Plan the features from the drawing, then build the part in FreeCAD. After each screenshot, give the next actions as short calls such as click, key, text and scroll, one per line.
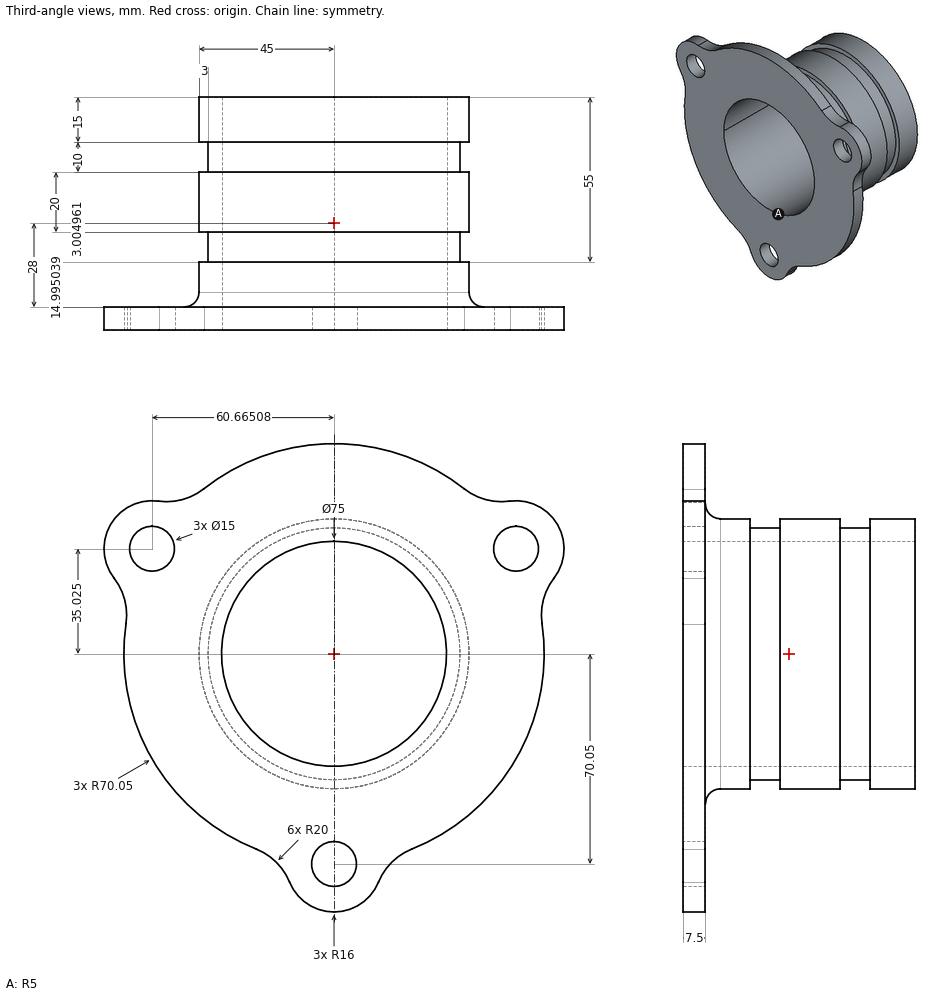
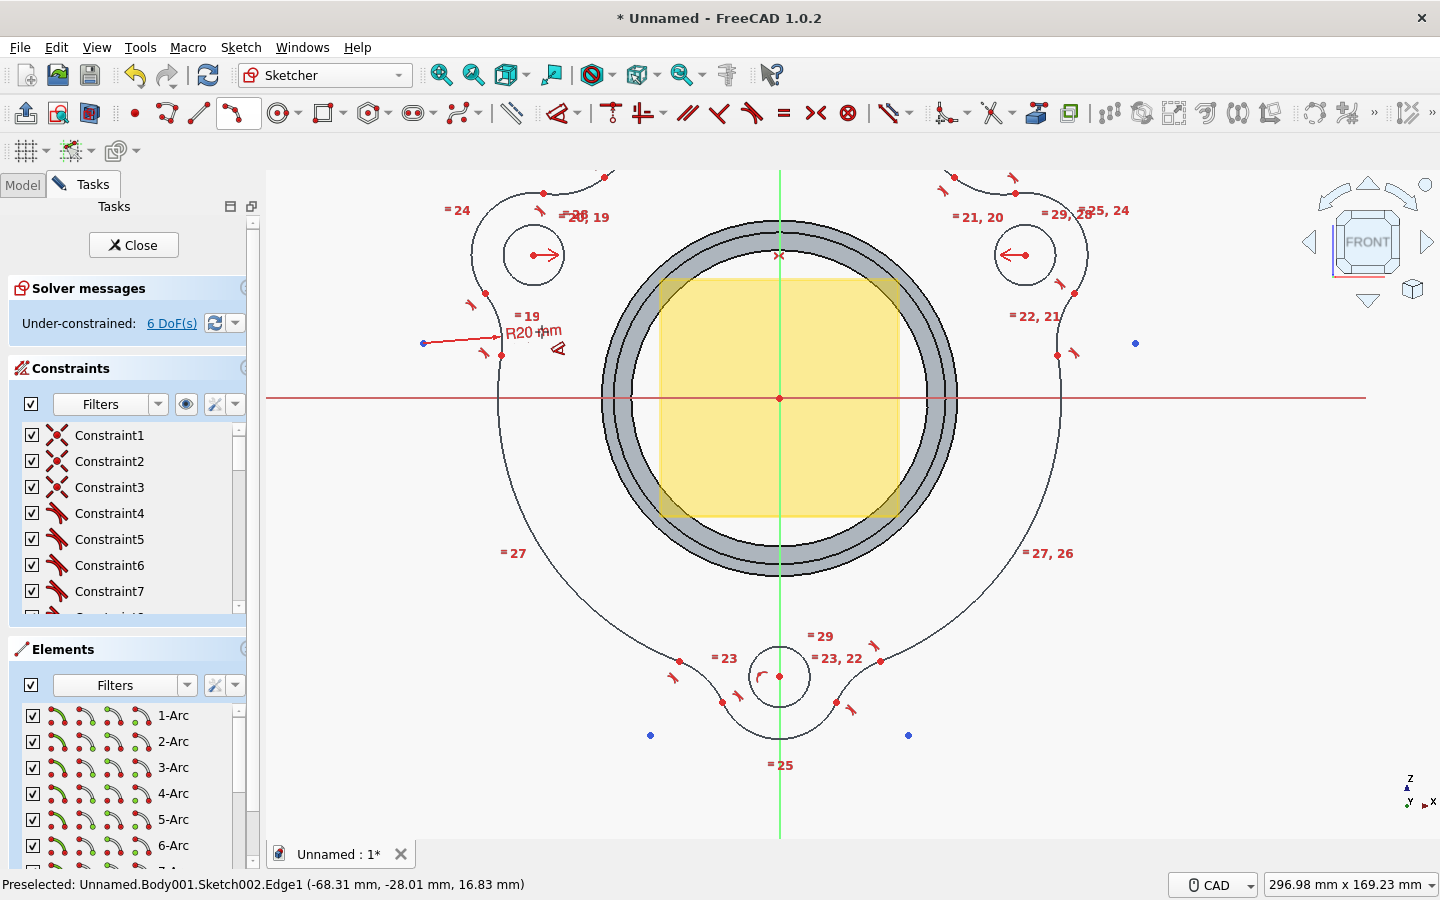
click(500, 202)
click(451, 209)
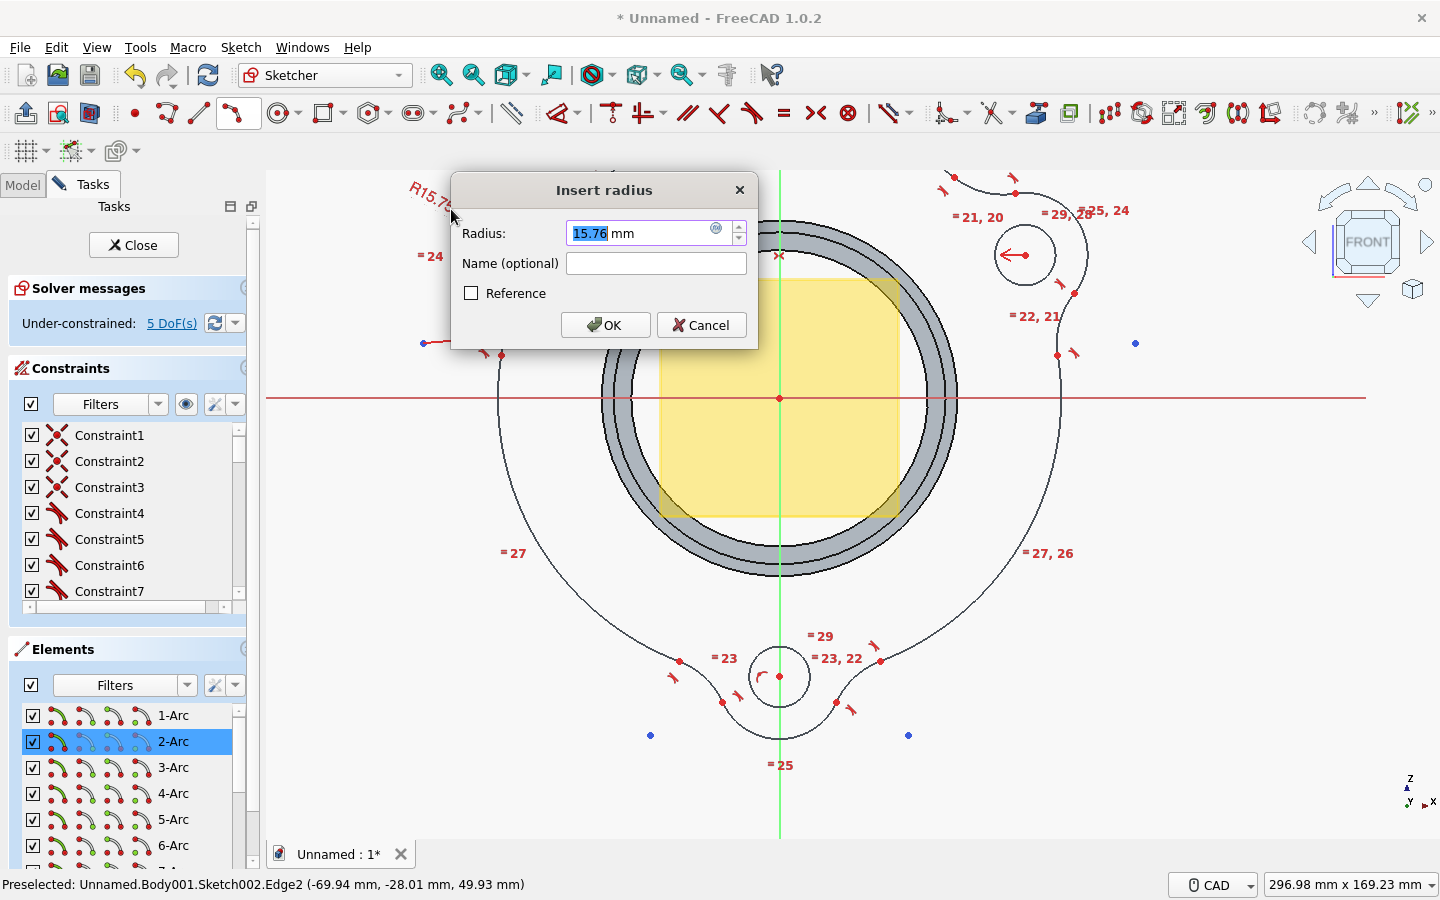
text(16)
key(Return)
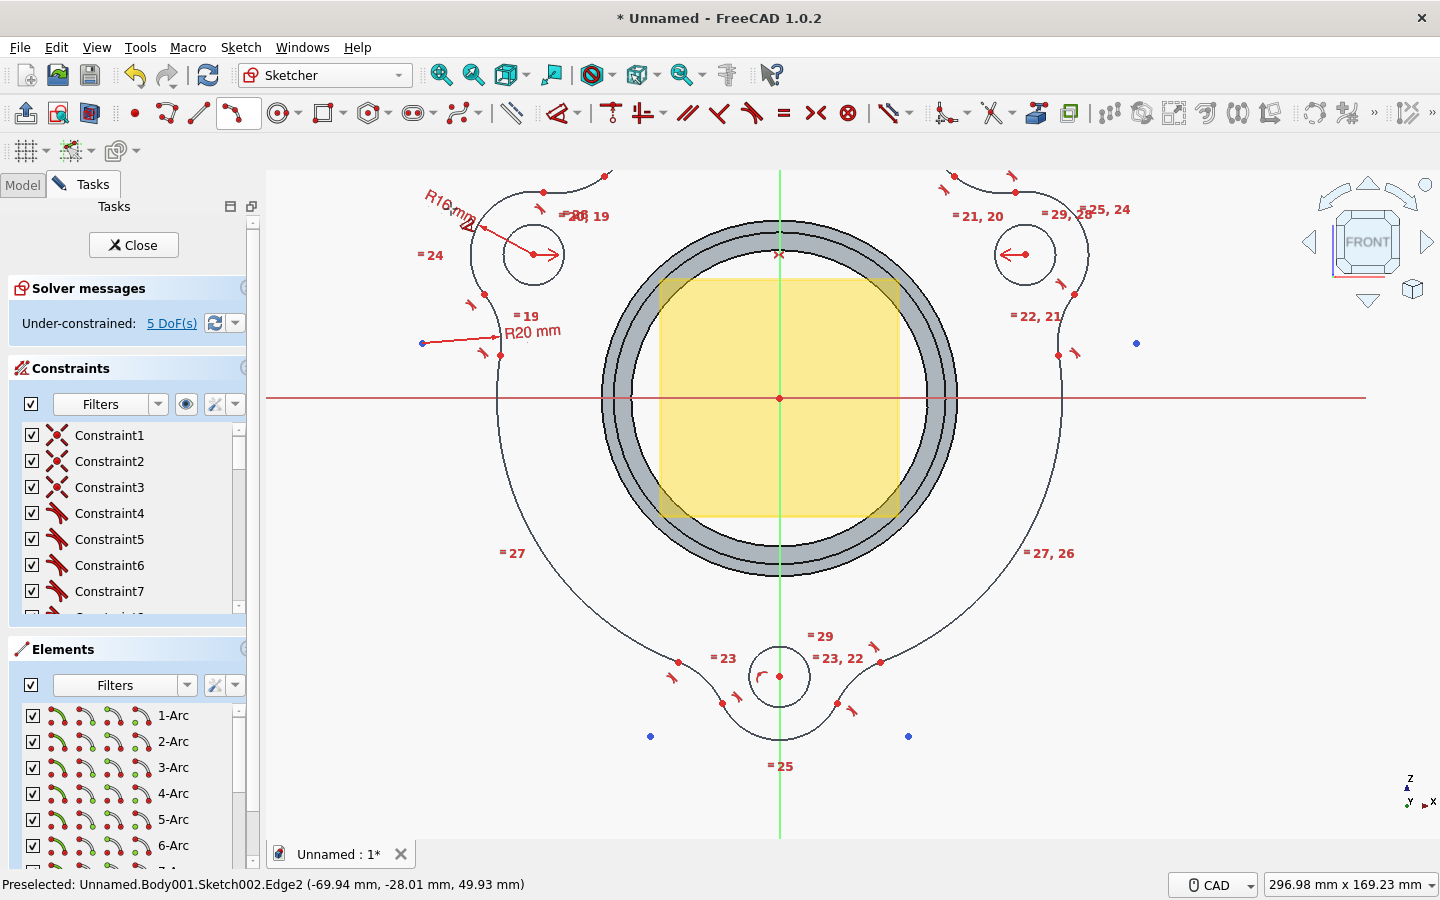
scroll(795, 656, down, 2)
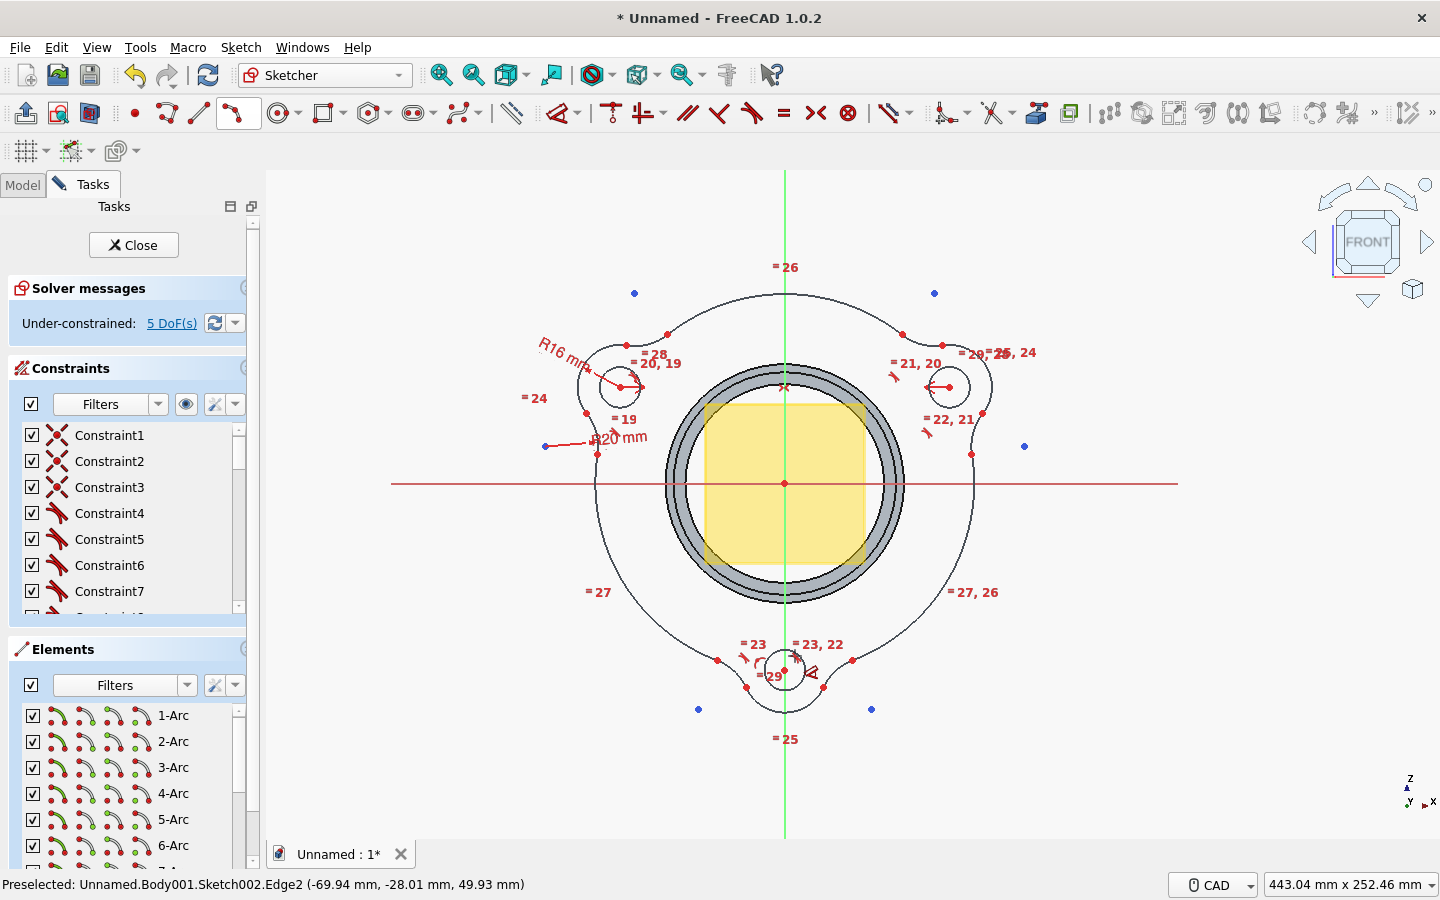
click(835, 301)
click(843, 270)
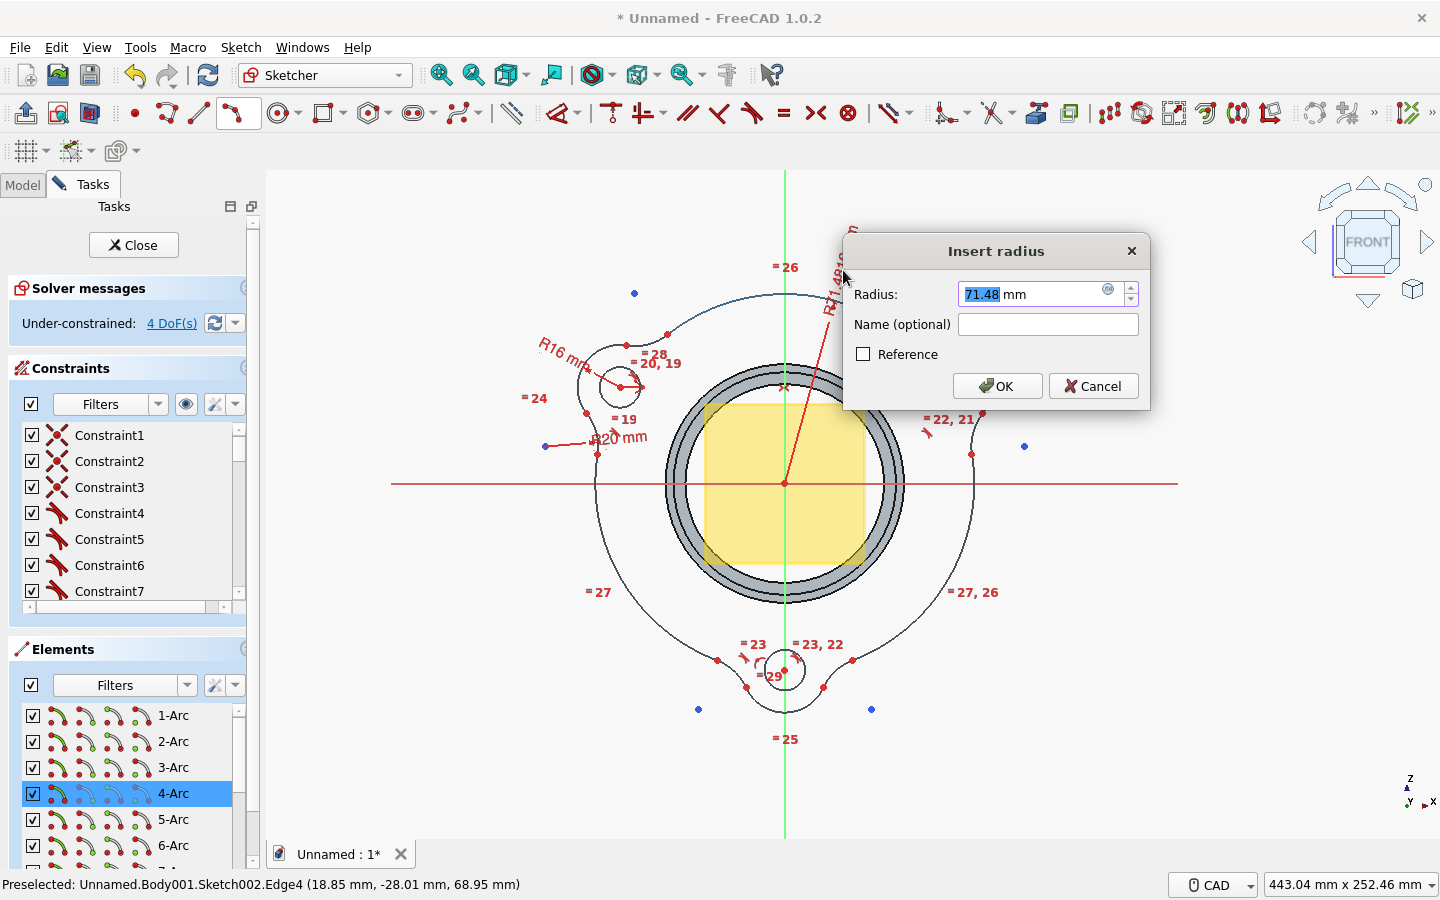
text(70.05)
key(Return)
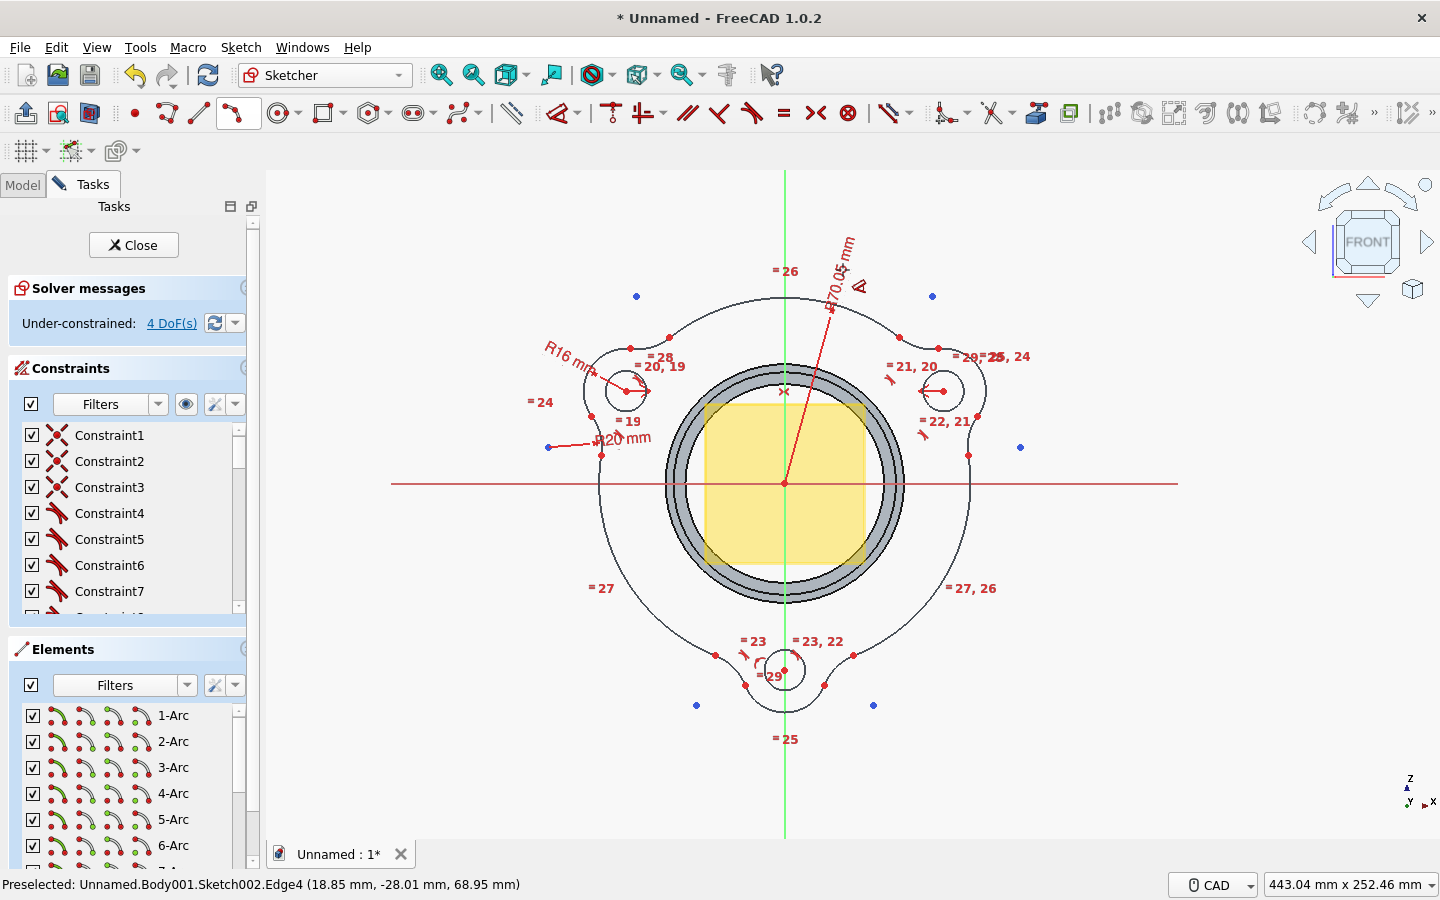
click(640, 377)
click(676, 376)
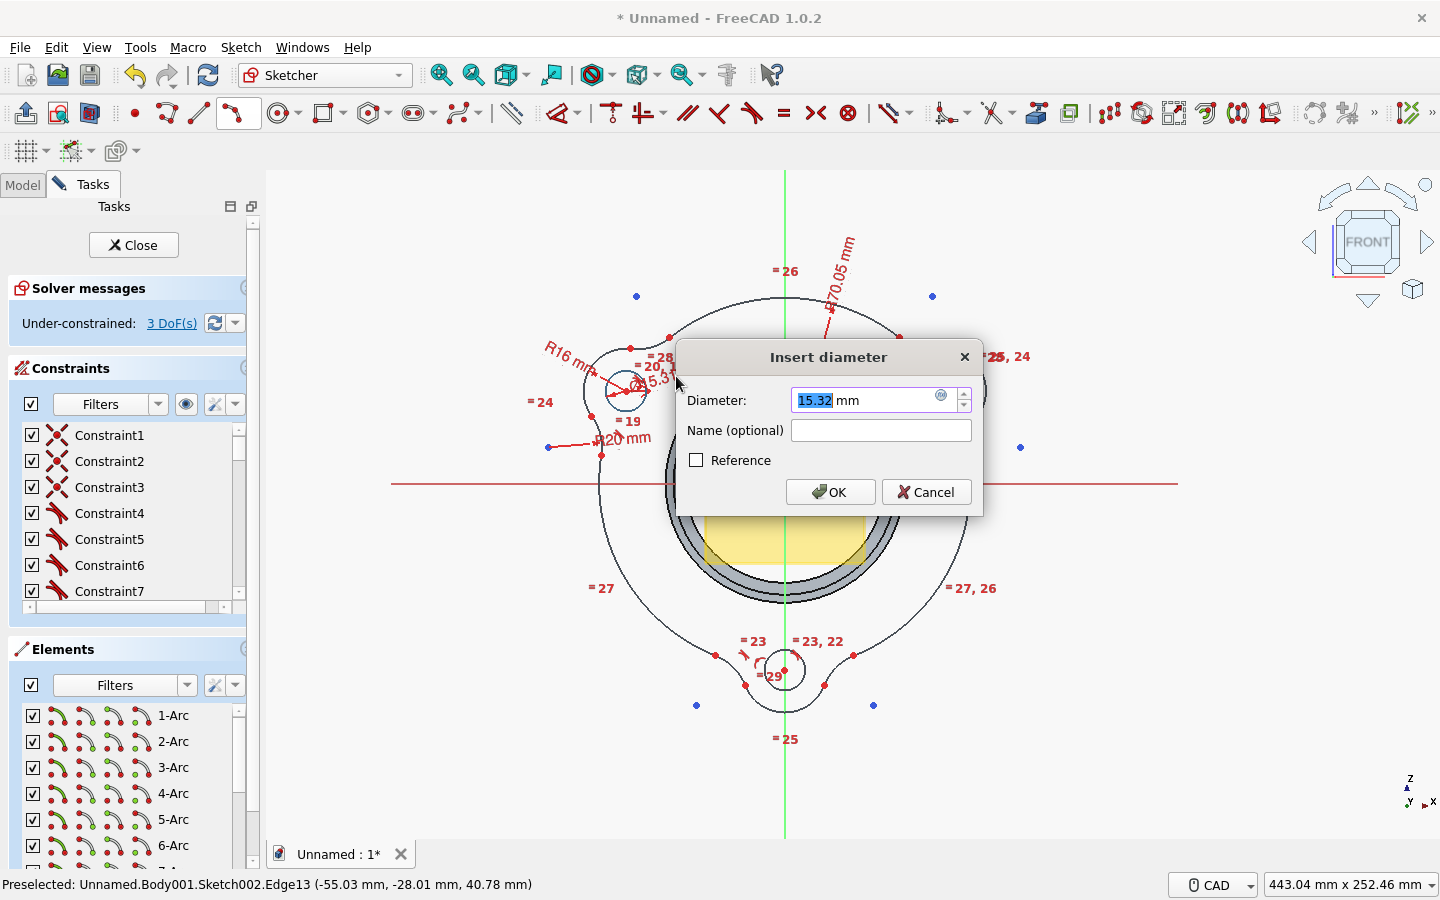
text(15)
key(Return)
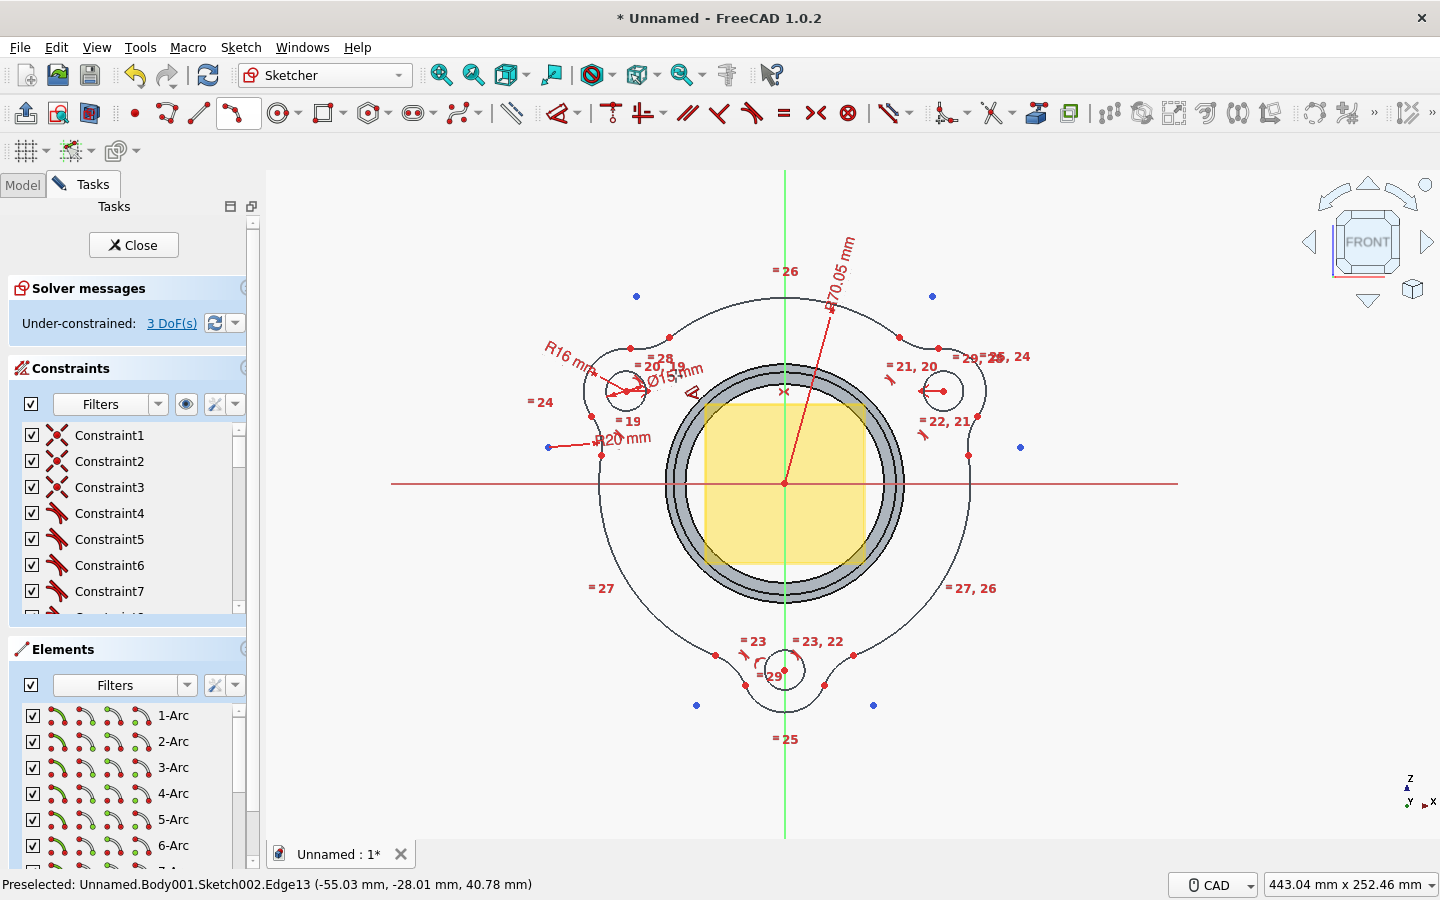
click(785, 670)
click(819, 577)